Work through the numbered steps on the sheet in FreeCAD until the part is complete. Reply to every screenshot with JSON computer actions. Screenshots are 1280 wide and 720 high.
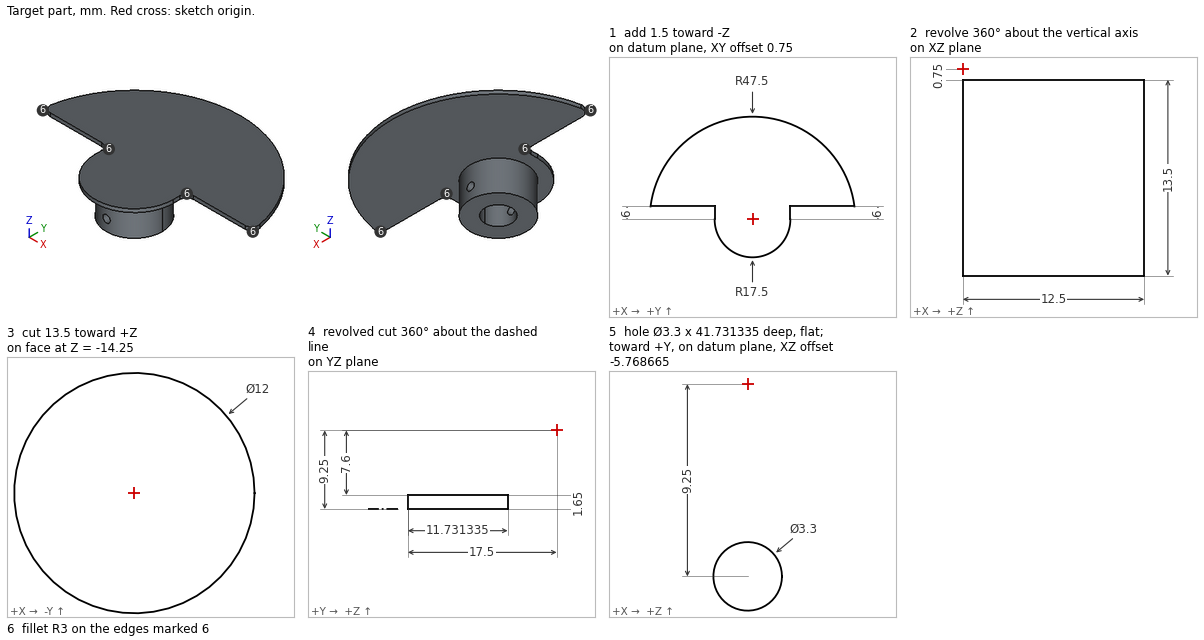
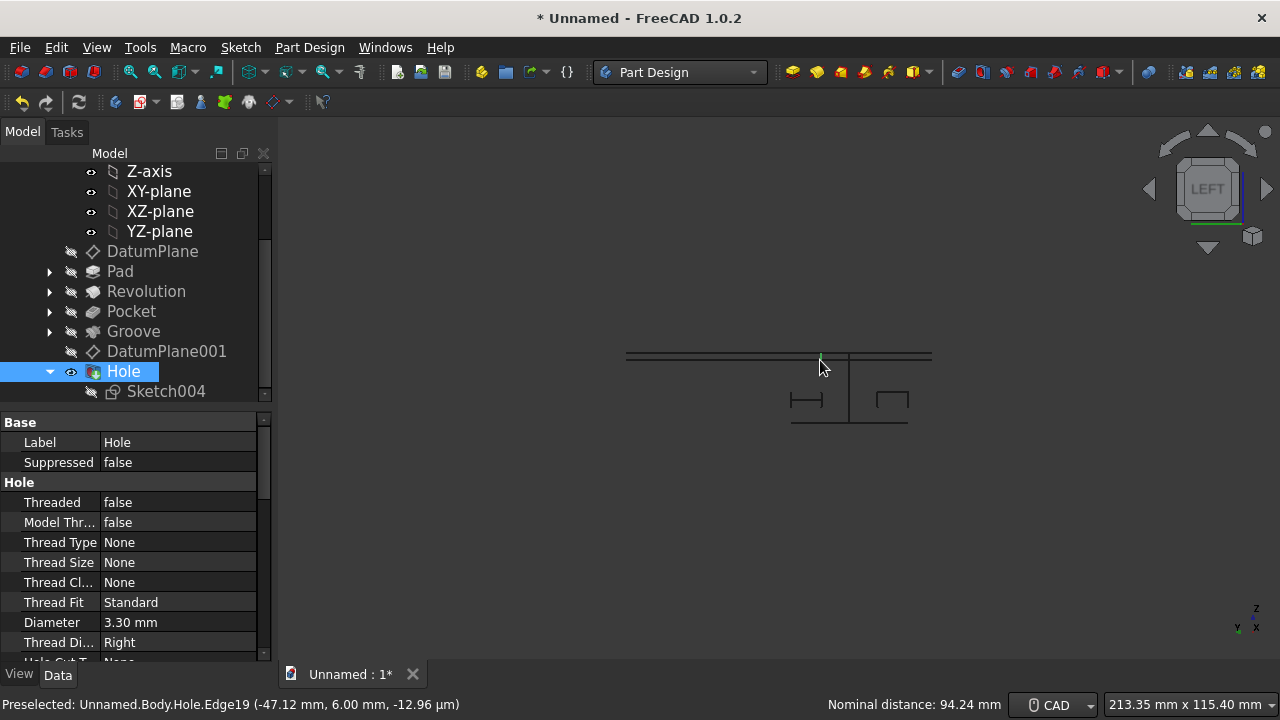
{"action": "key", "text": "0"}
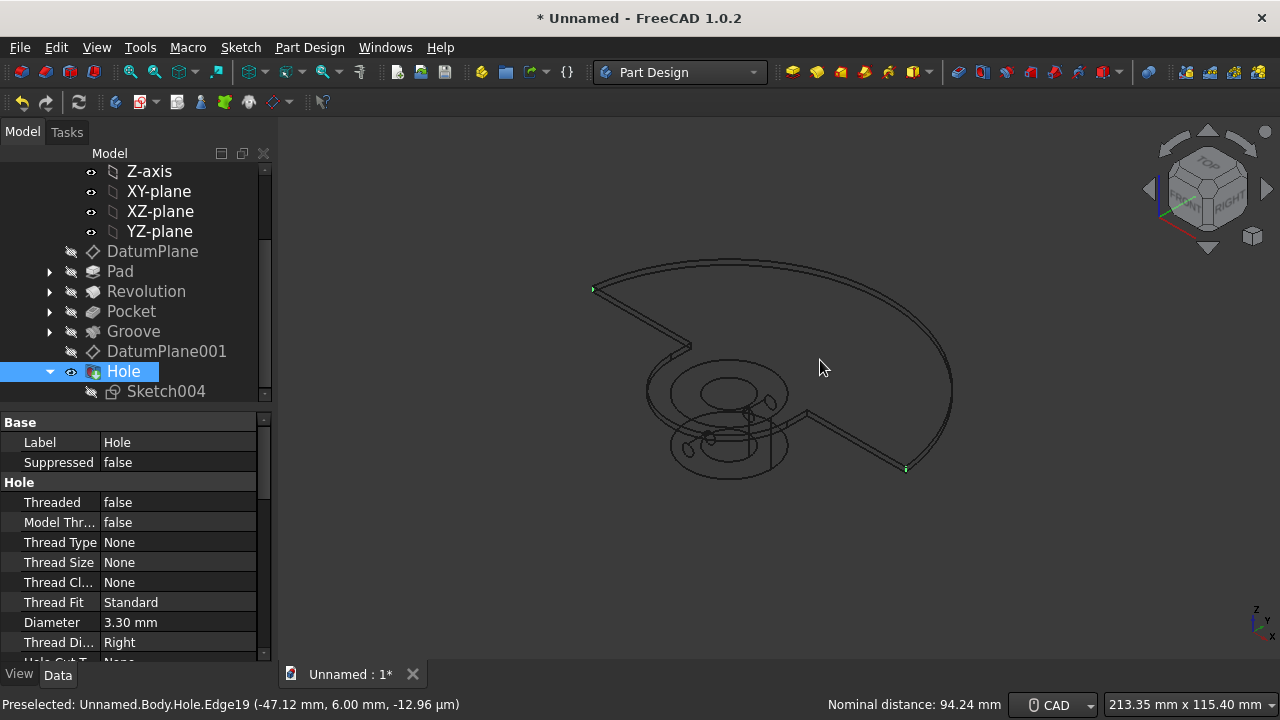
{"action": "scroll", "coordinate": [691, 345], "scroll_direction": "up", "scroll_amount": 9}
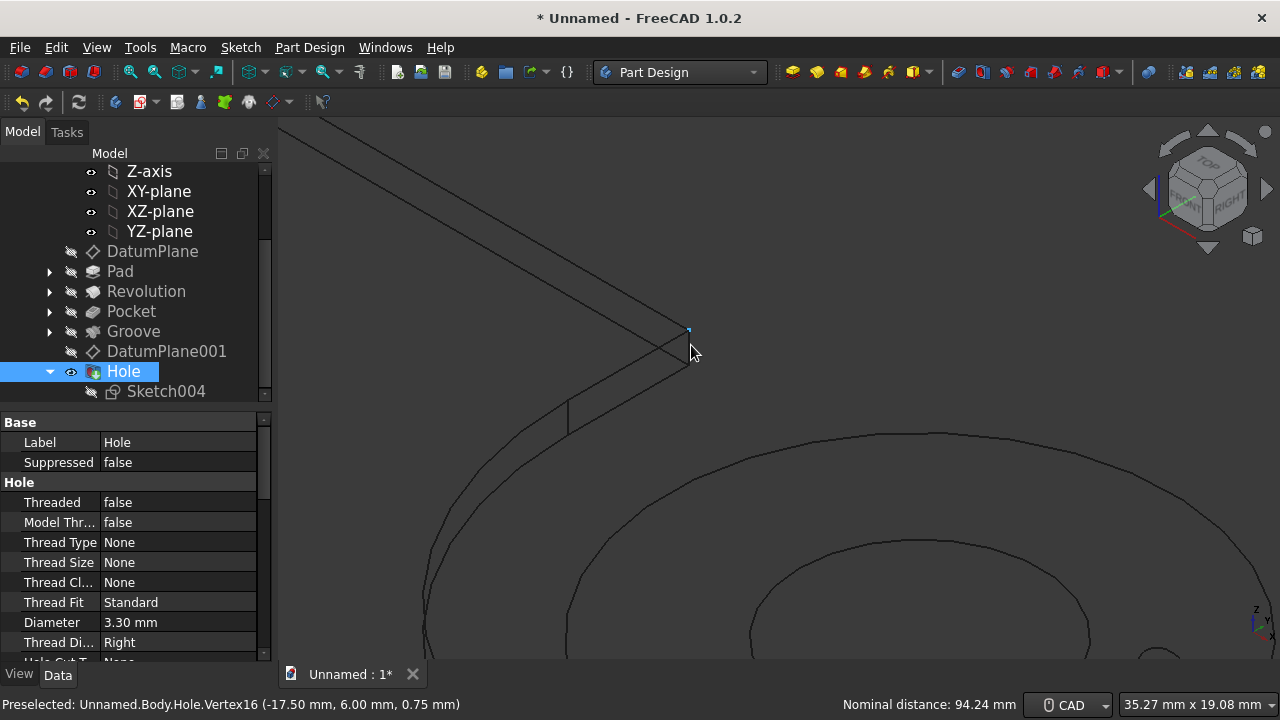
{"action": "left_click", "coordinate": [689, 347], "text": "ctrl"}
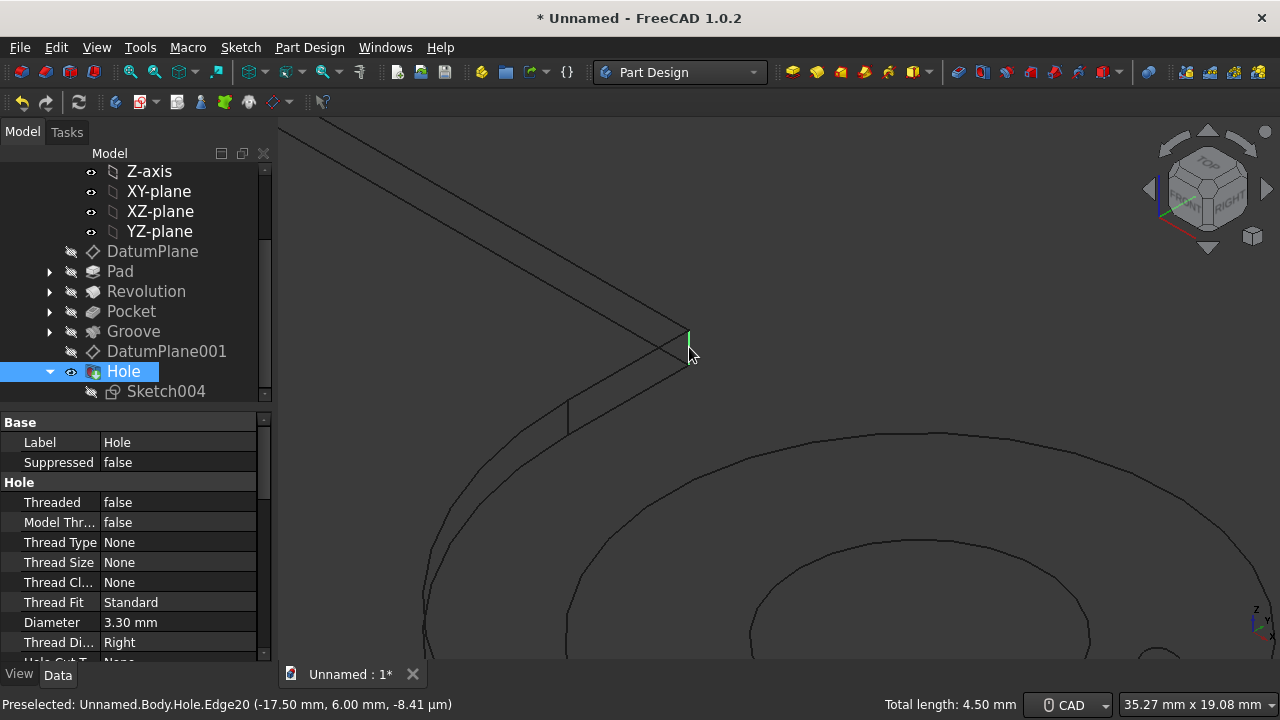
{"action": "key", "text": "v f"}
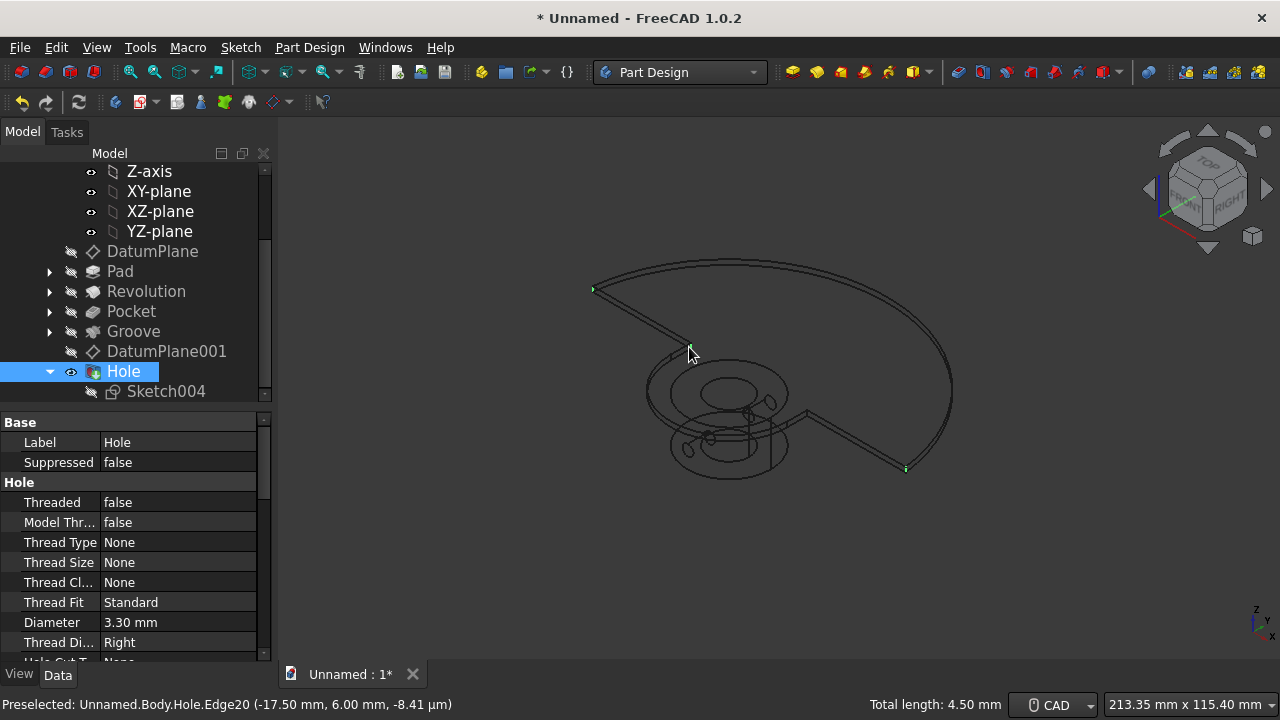
{"action": "key", "text": "2"}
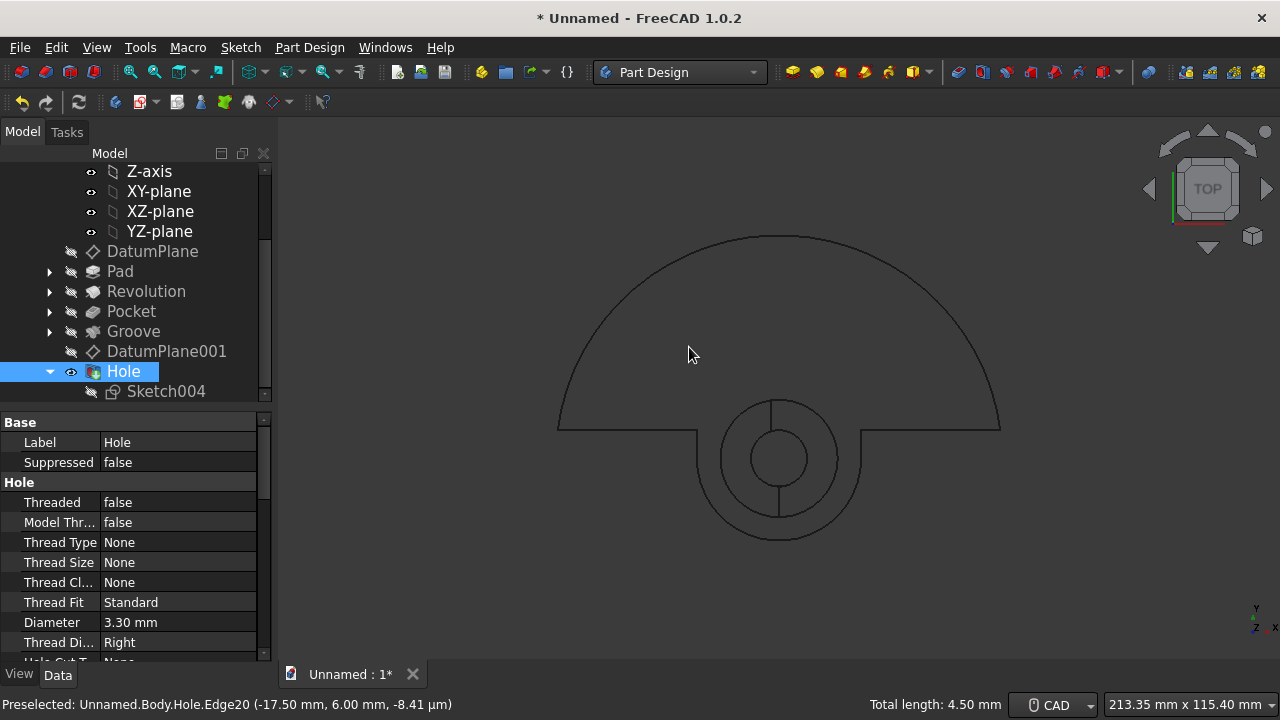
{"action": "scroll", "coordinate": [861, 429], "scroll_direction": "up", "scroll_amount": 9}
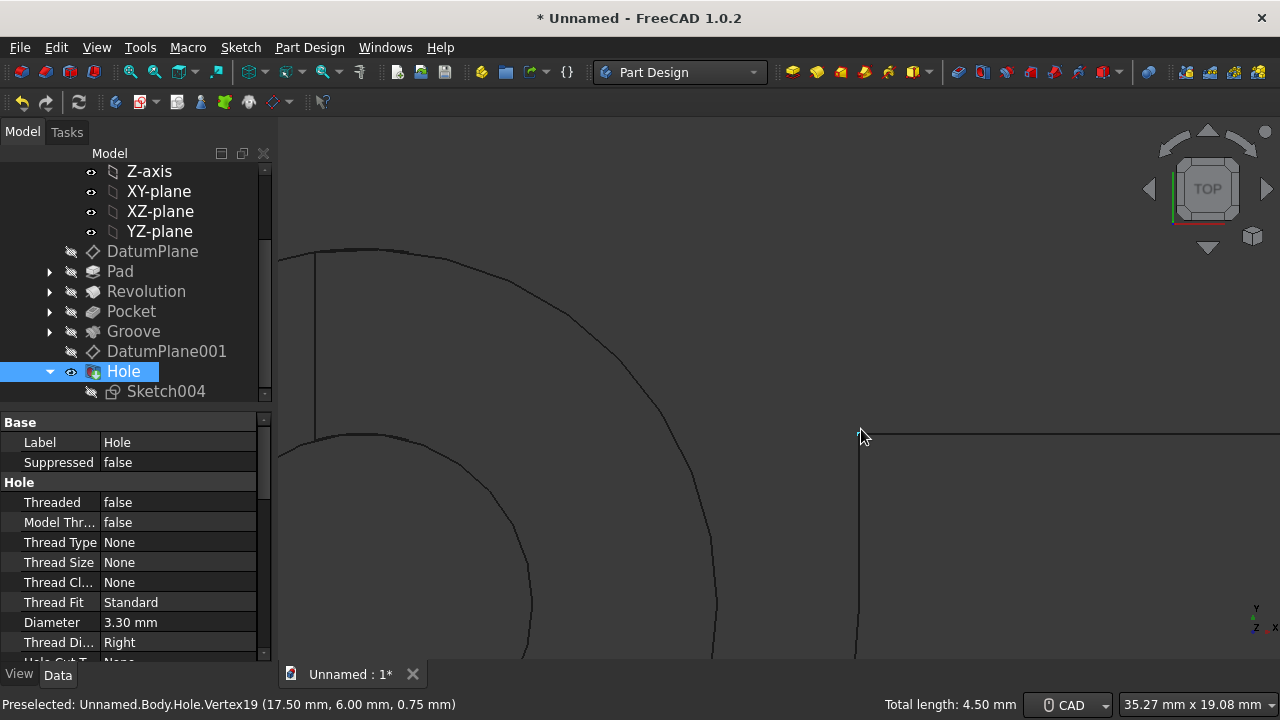
{"action": "key", "text": "v f"}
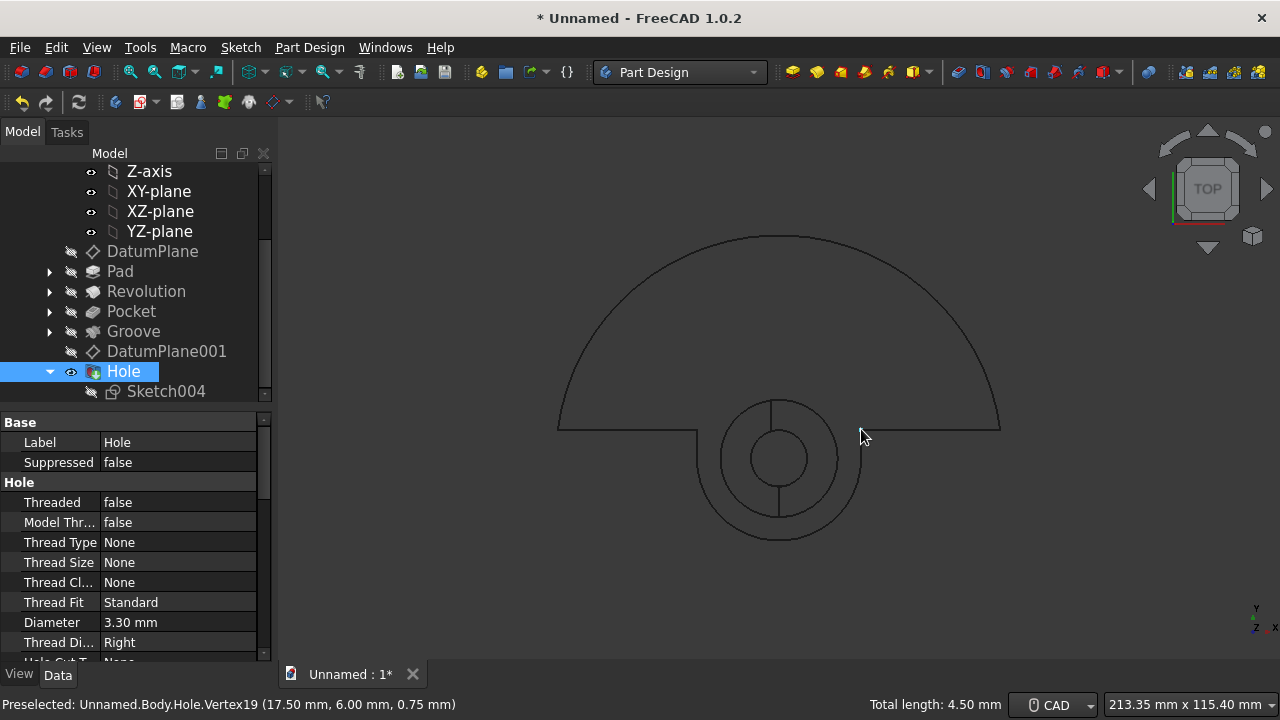
{"action": "key", "text": "1"}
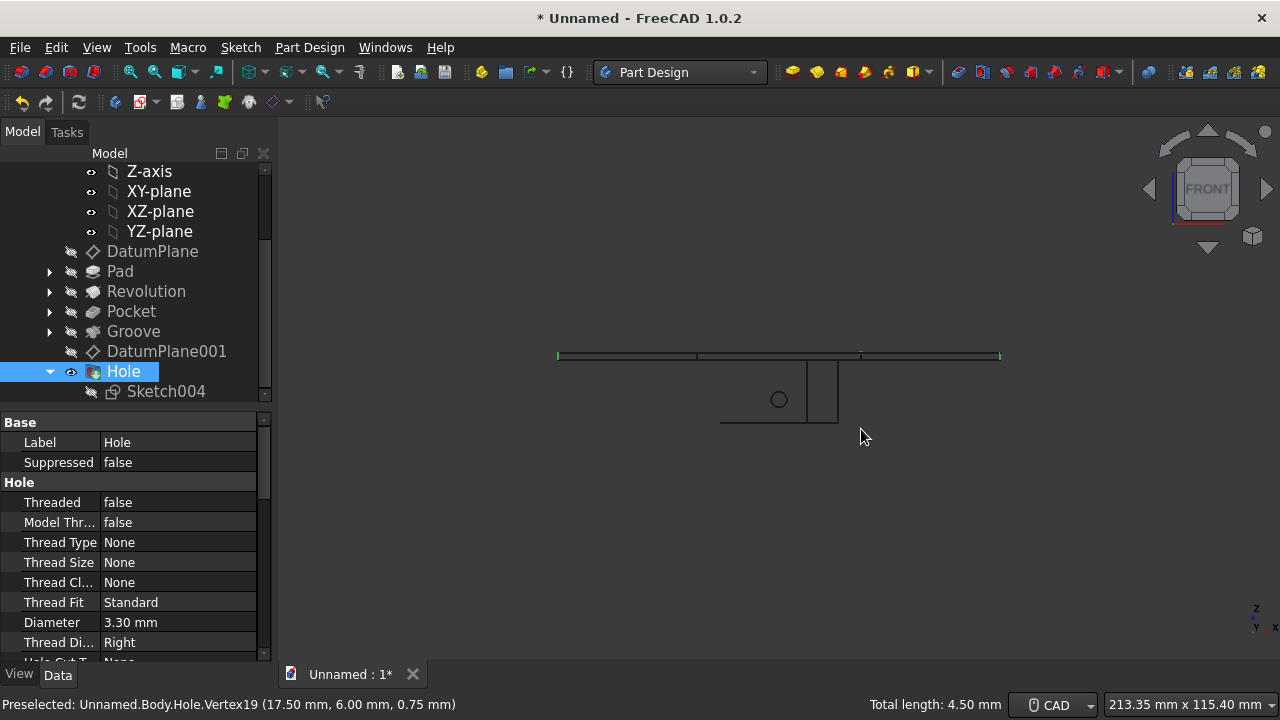
{"action": "key", "text": "v f"}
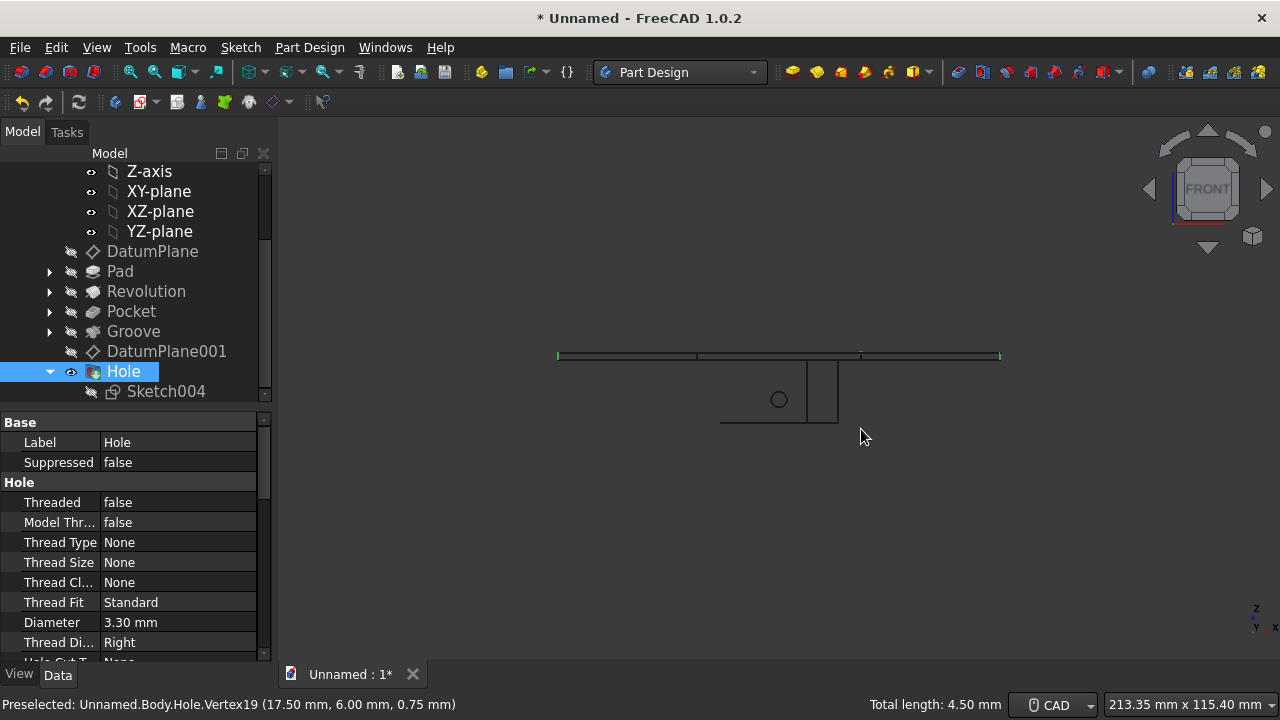
{"action": "scroll", "coordinate": [861, 355], "scroll_direction": "up", "scroll_amount": 9}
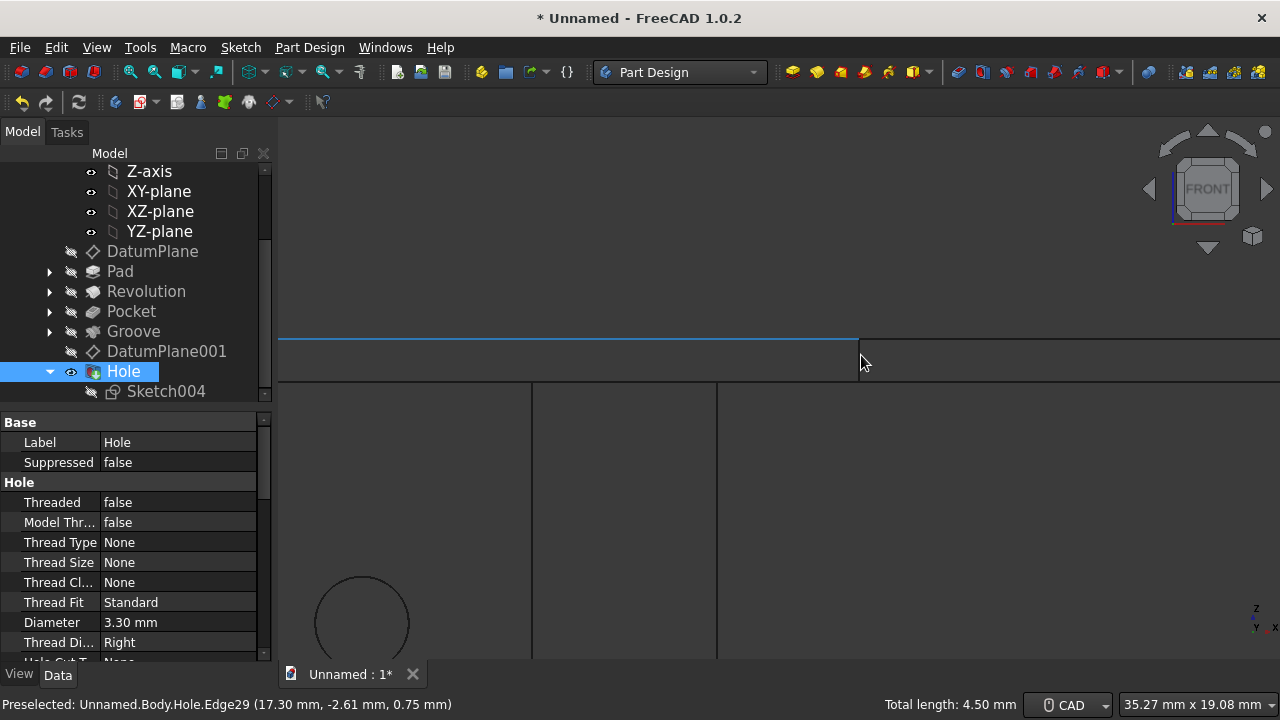
{"action": "key", "text": "v f"}